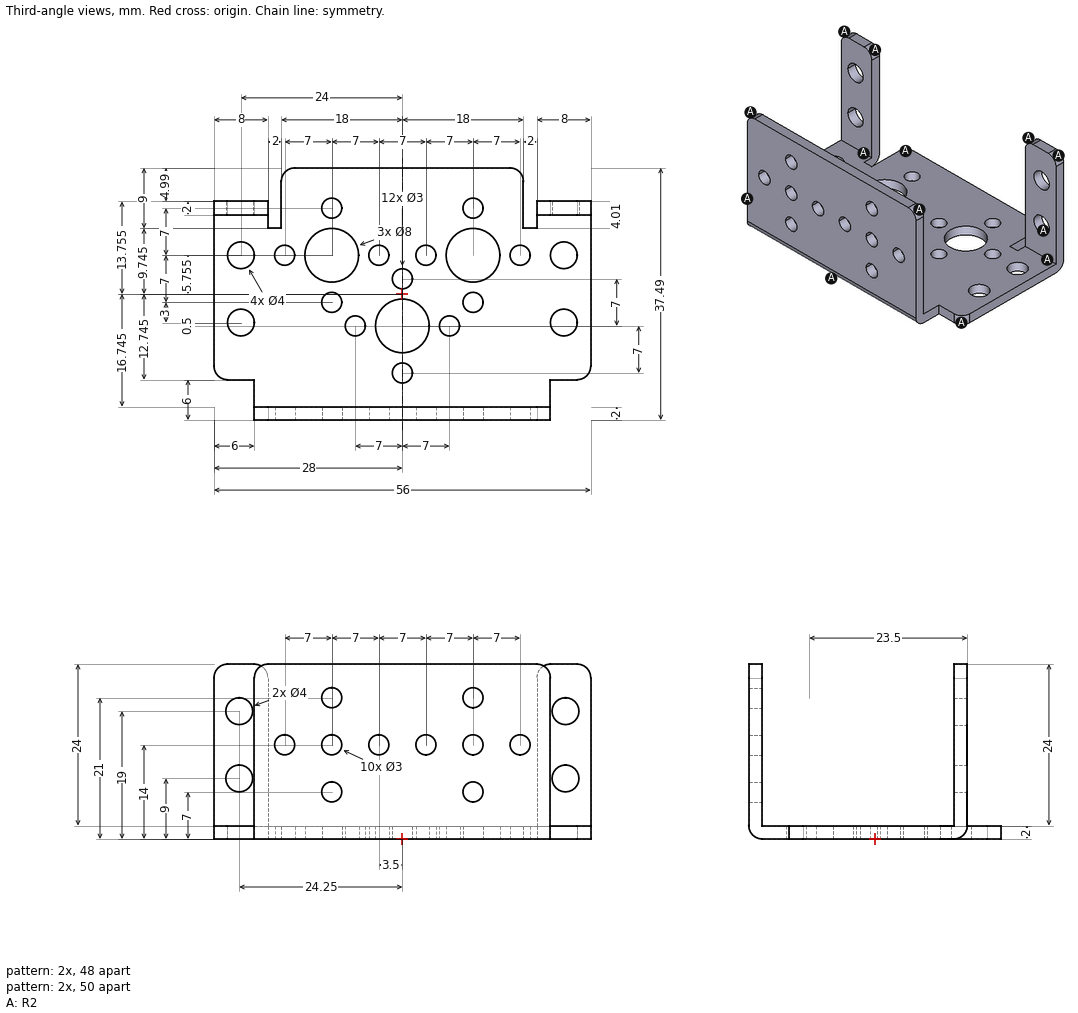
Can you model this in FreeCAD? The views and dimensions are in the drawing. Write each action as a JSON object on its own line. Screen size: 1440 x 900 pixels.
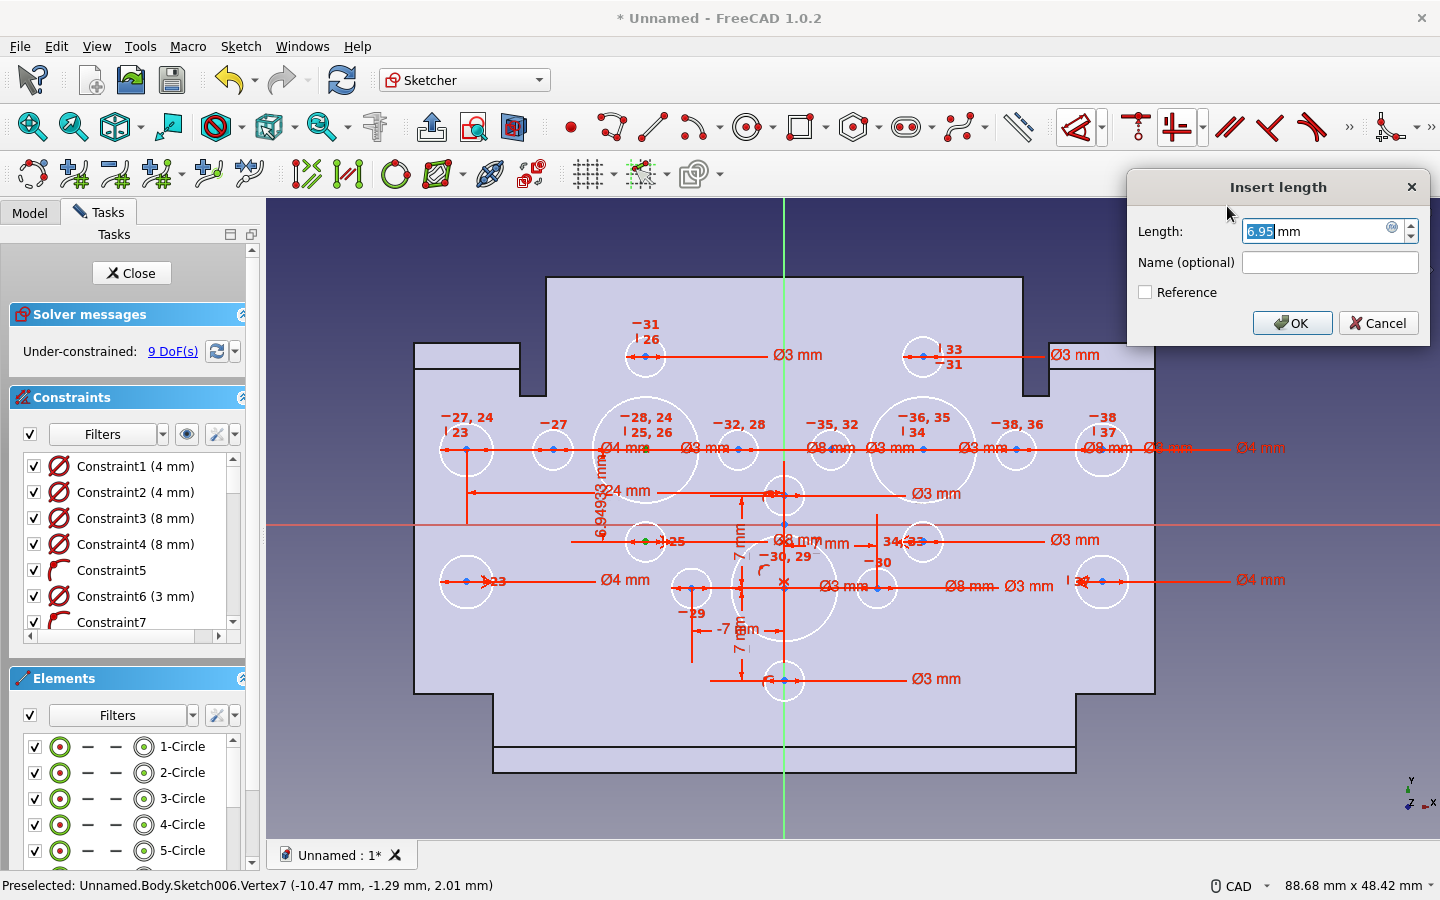
{"action": "type", "text": "7"}
{"action": "key", "text": "Return"}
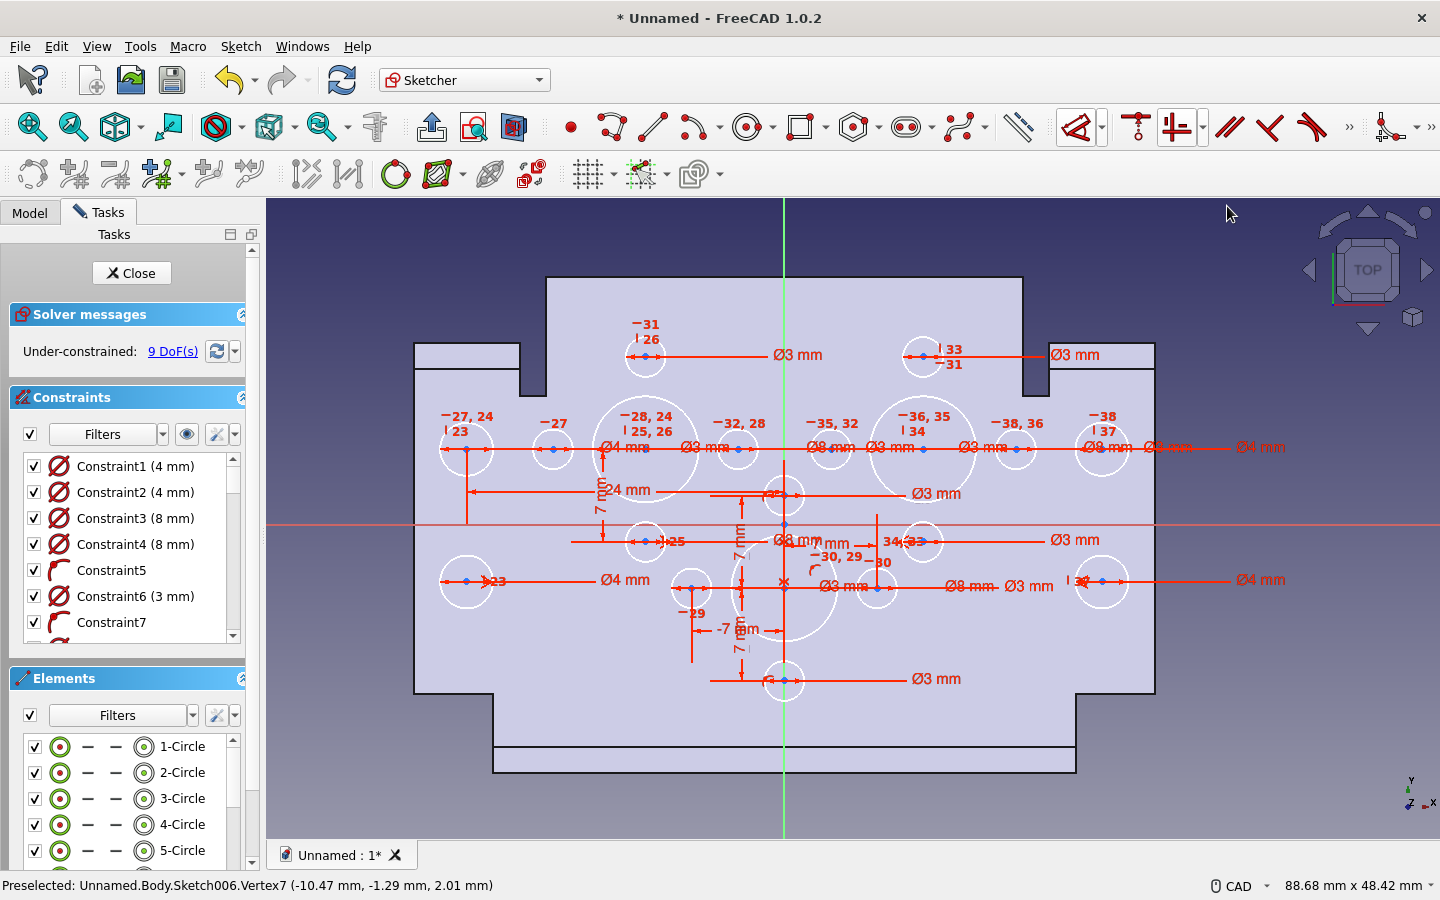
{"action": "left_click", "coordinate": [467, 582]}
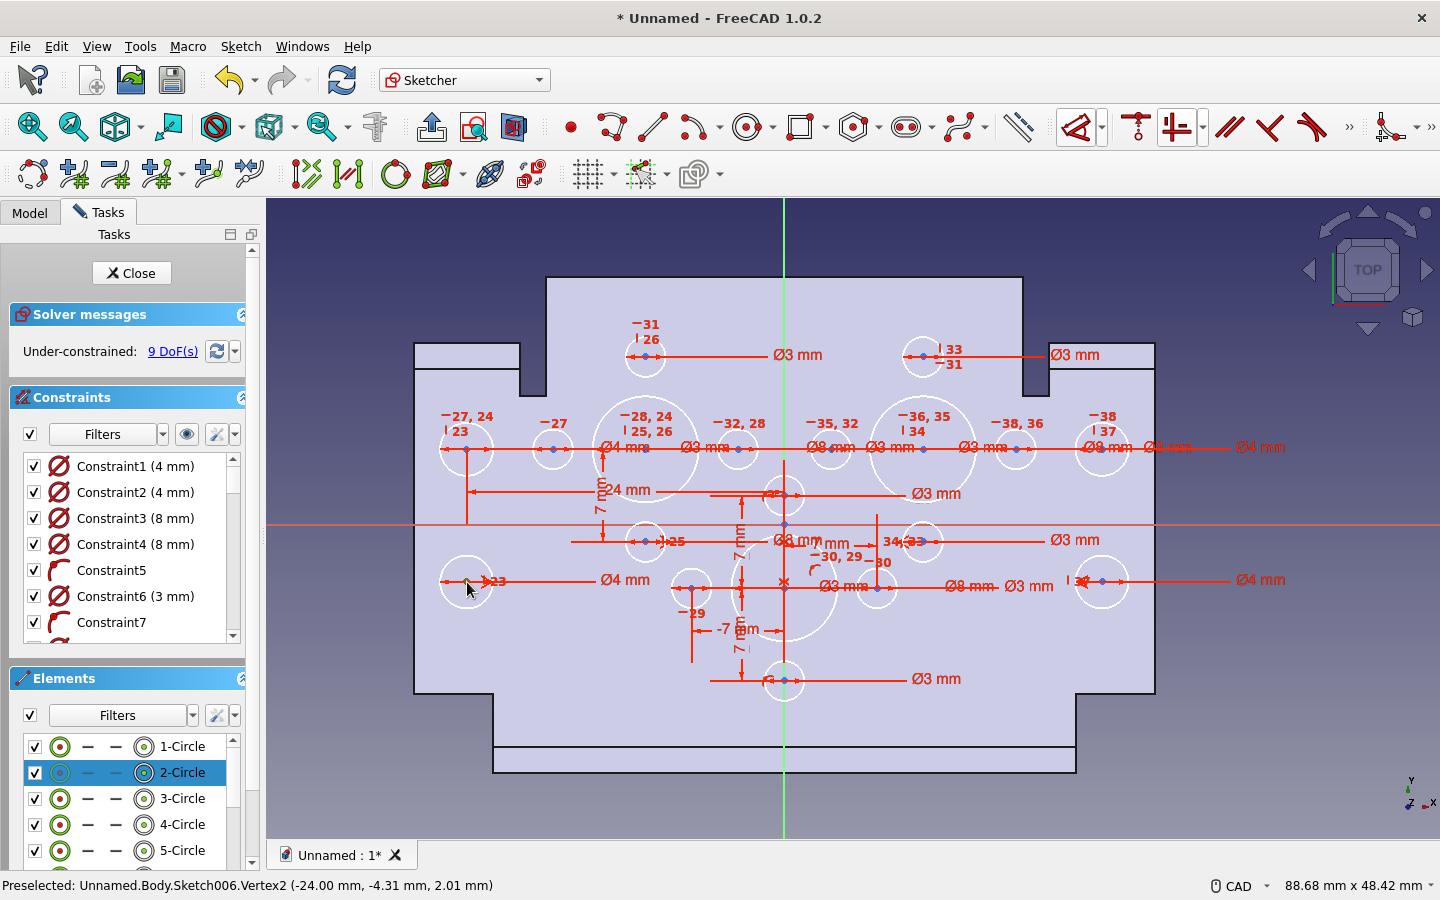
{"action": "left_click", "coordinate": [646, 542]}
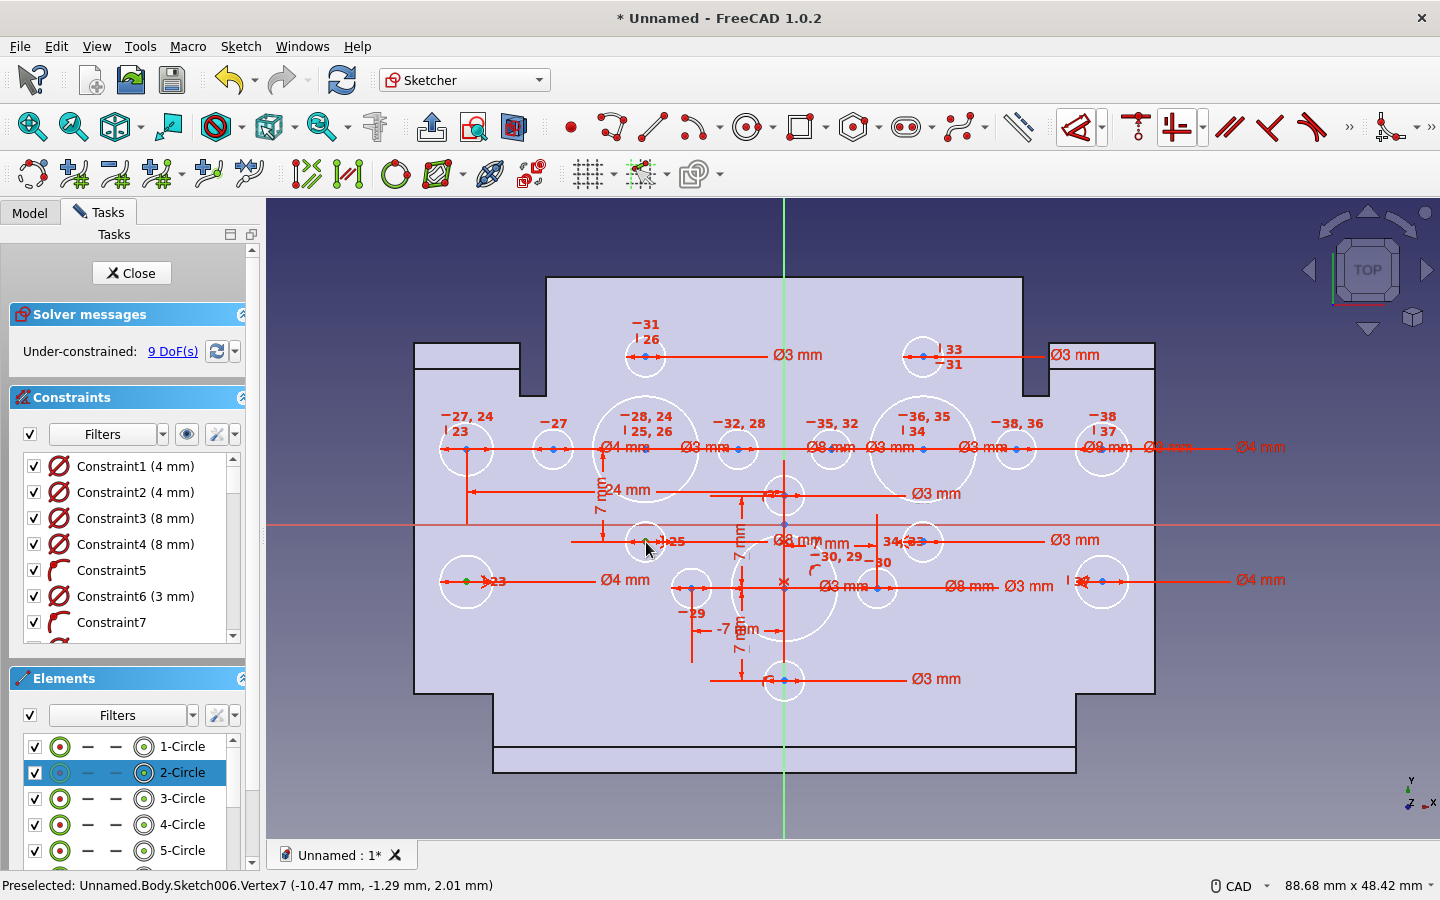
{"action": "key", "text": "i"}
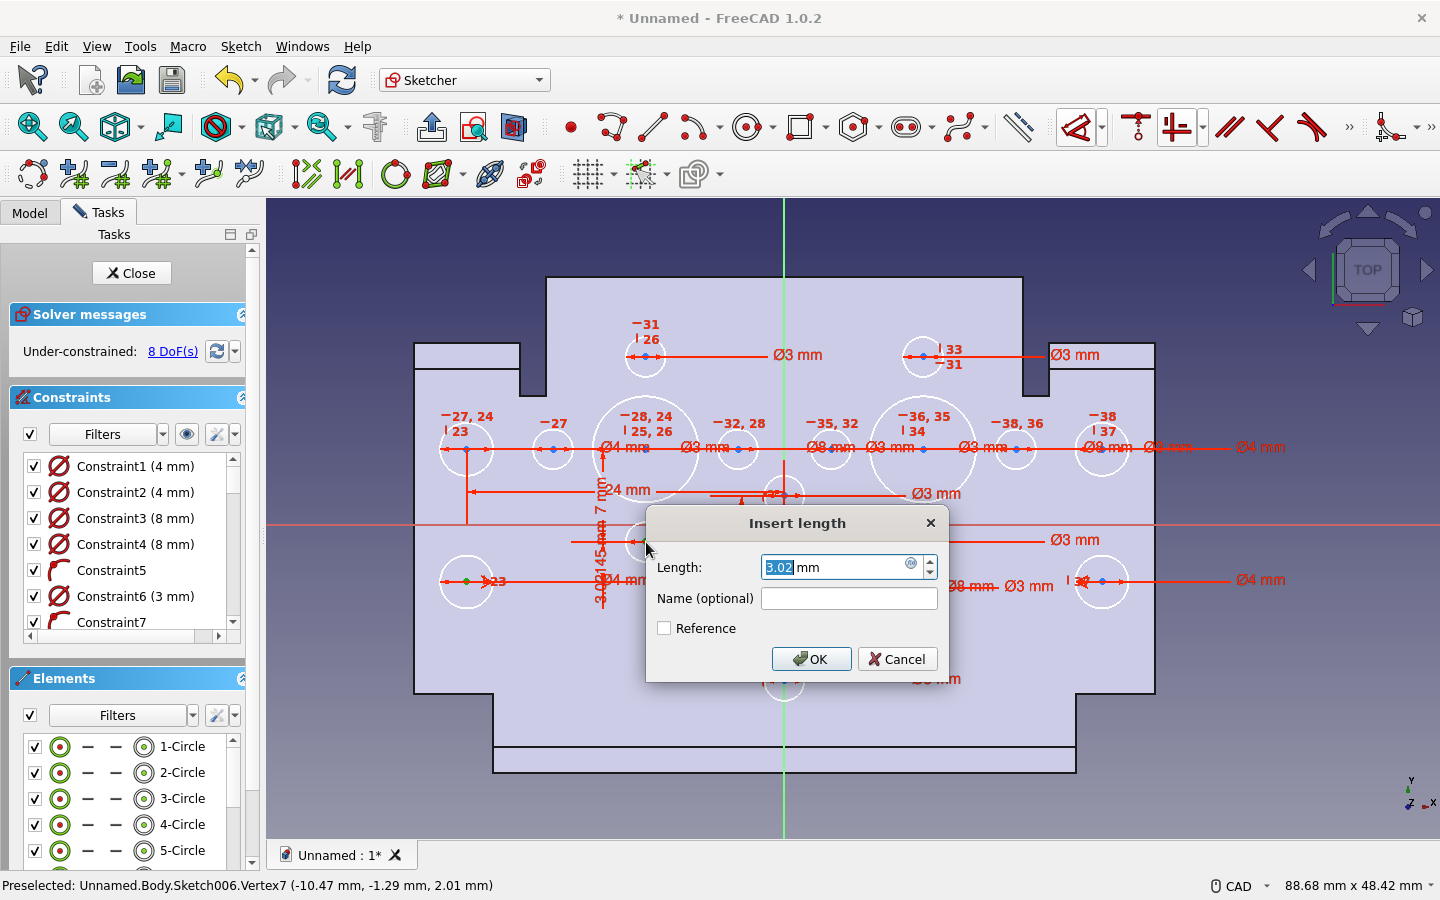
{"action": "type", "text": "3"}
{"action": "key", "text": "Return"}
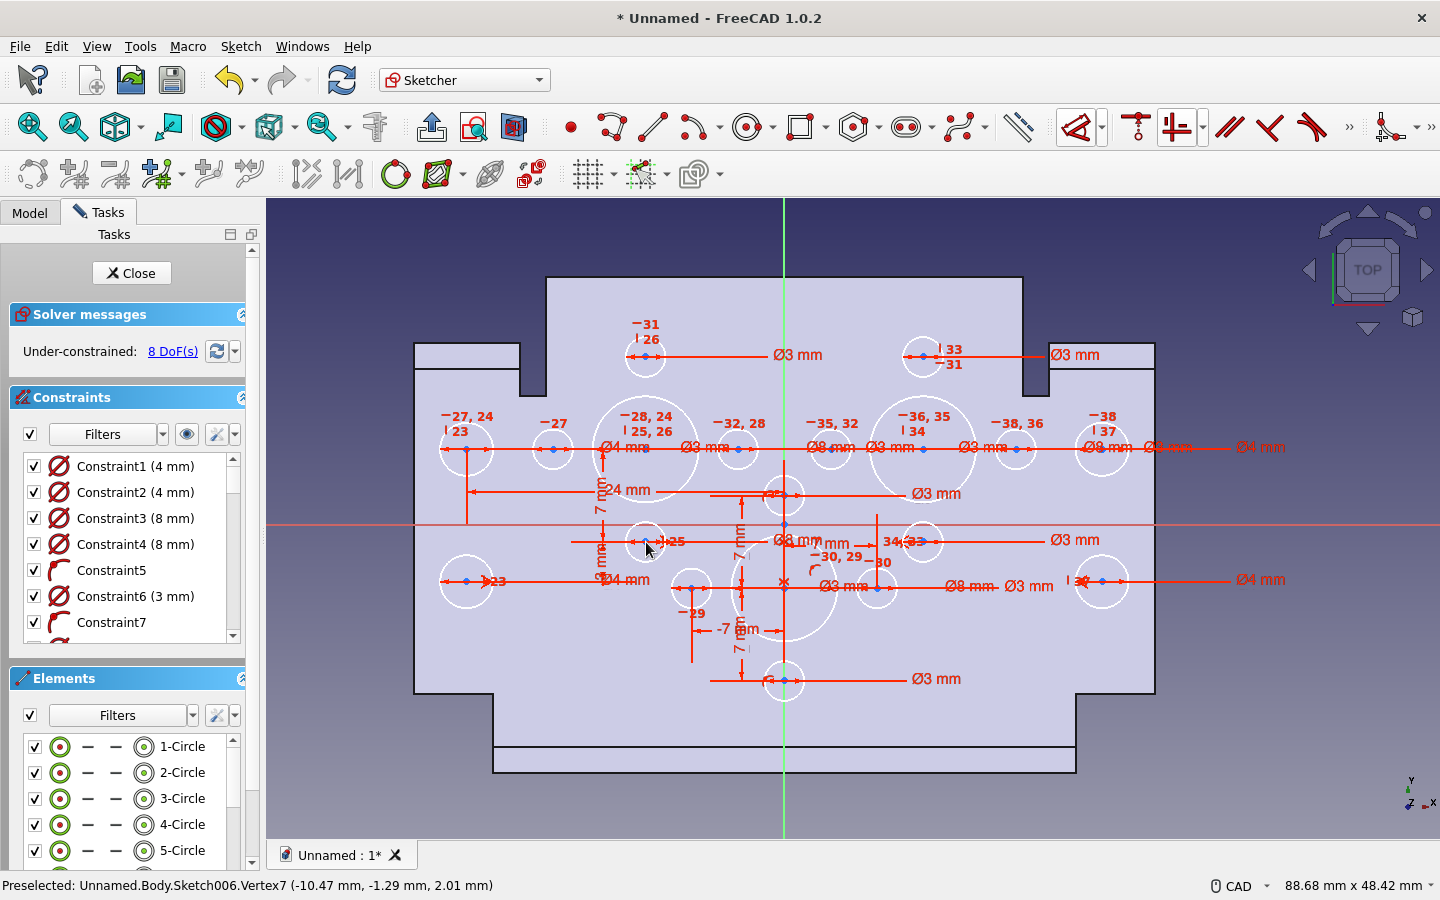
{"action": "left_click", "coordinate": [646, 449]}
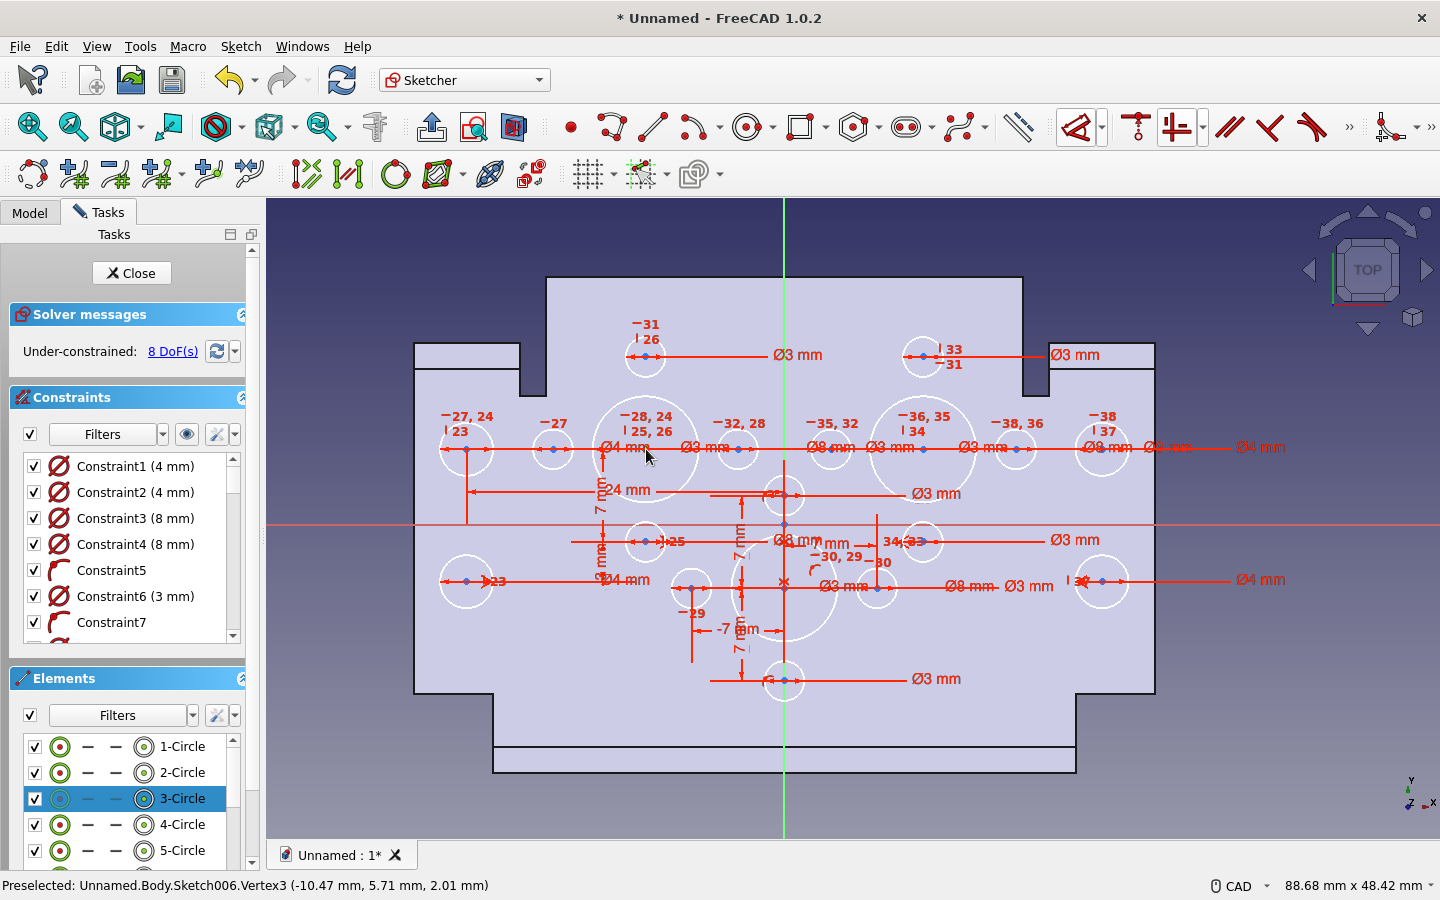
{"action": "left_click", "coordinate": [646, 357]}